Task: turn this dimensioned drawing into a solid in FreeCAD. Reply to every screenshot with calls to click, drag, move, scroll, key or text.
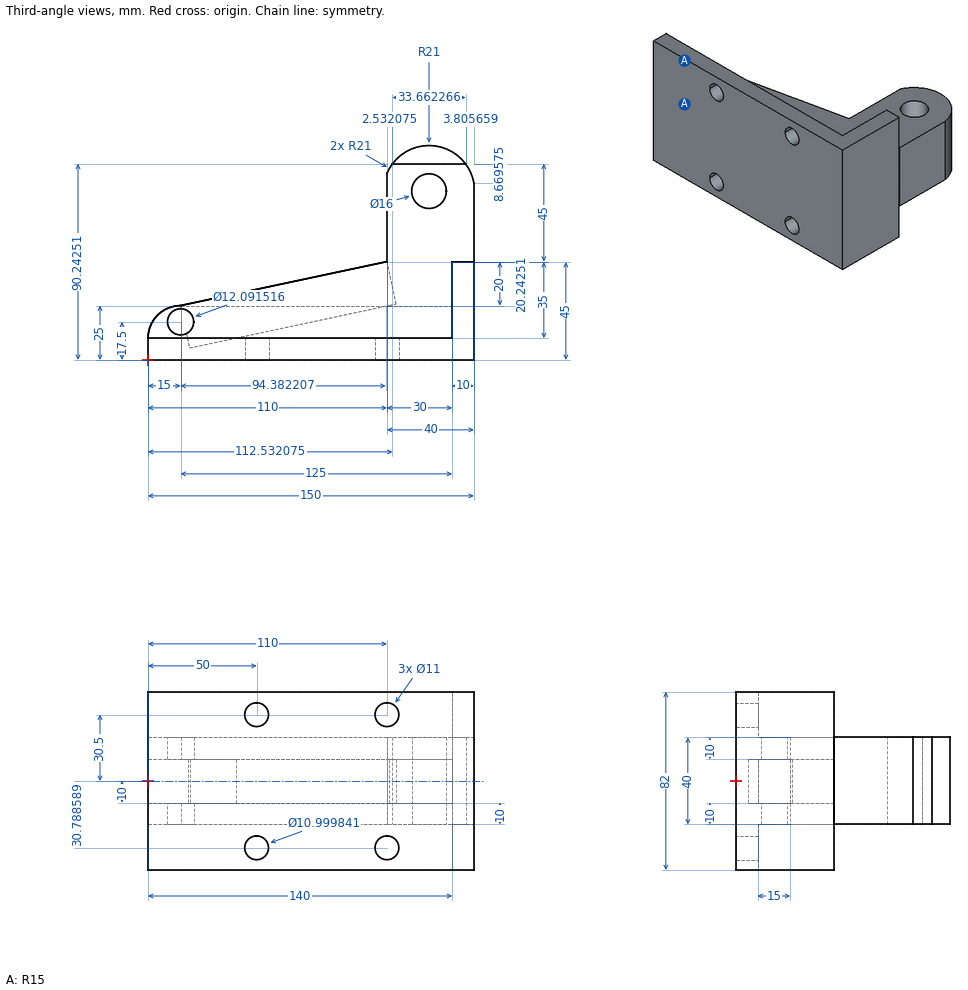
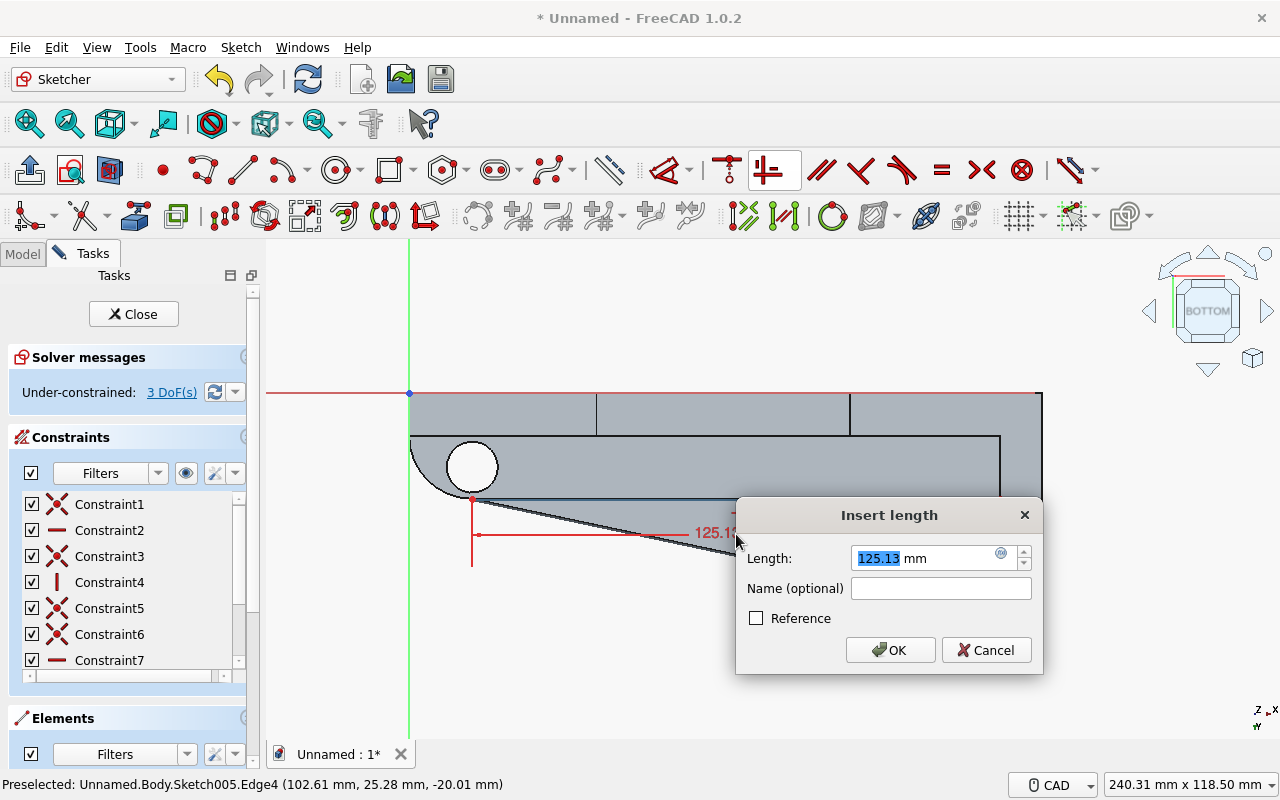
text(125)
key(Return)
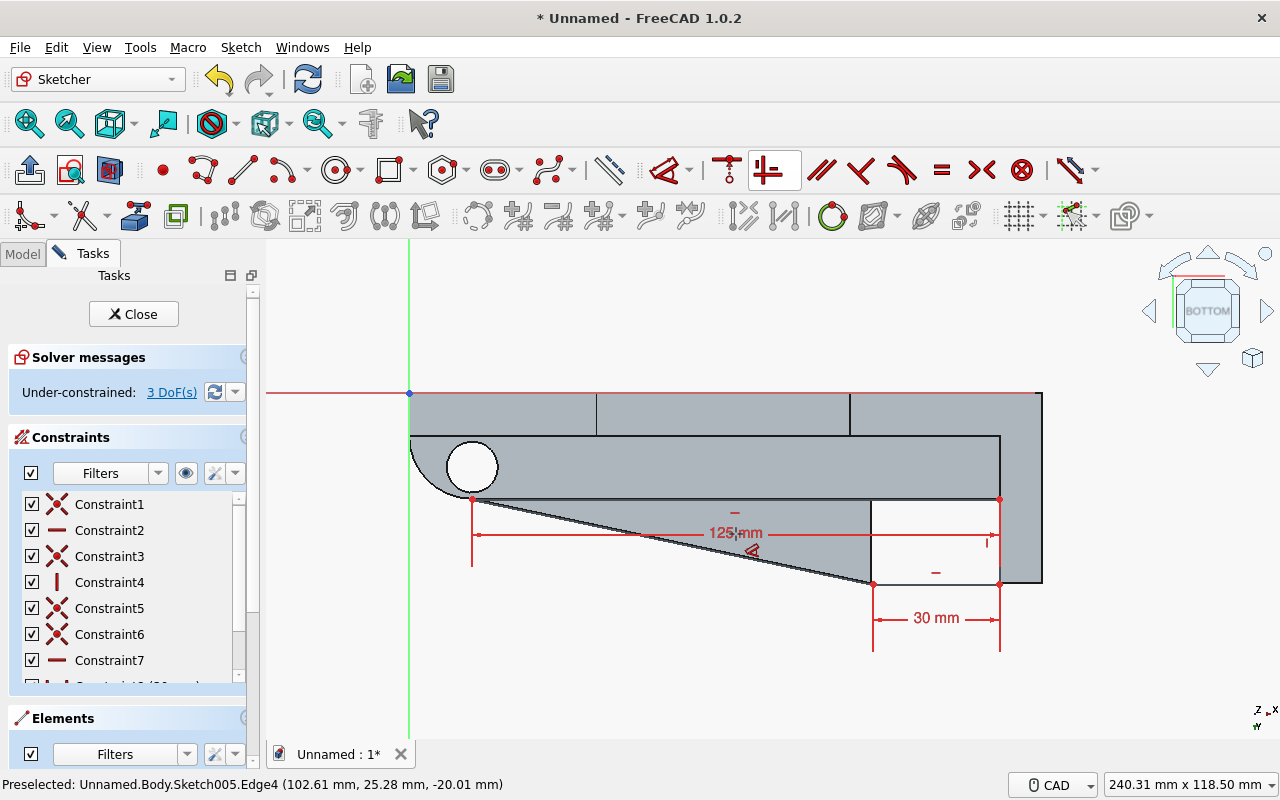
click(472, 500)
click(441, 359)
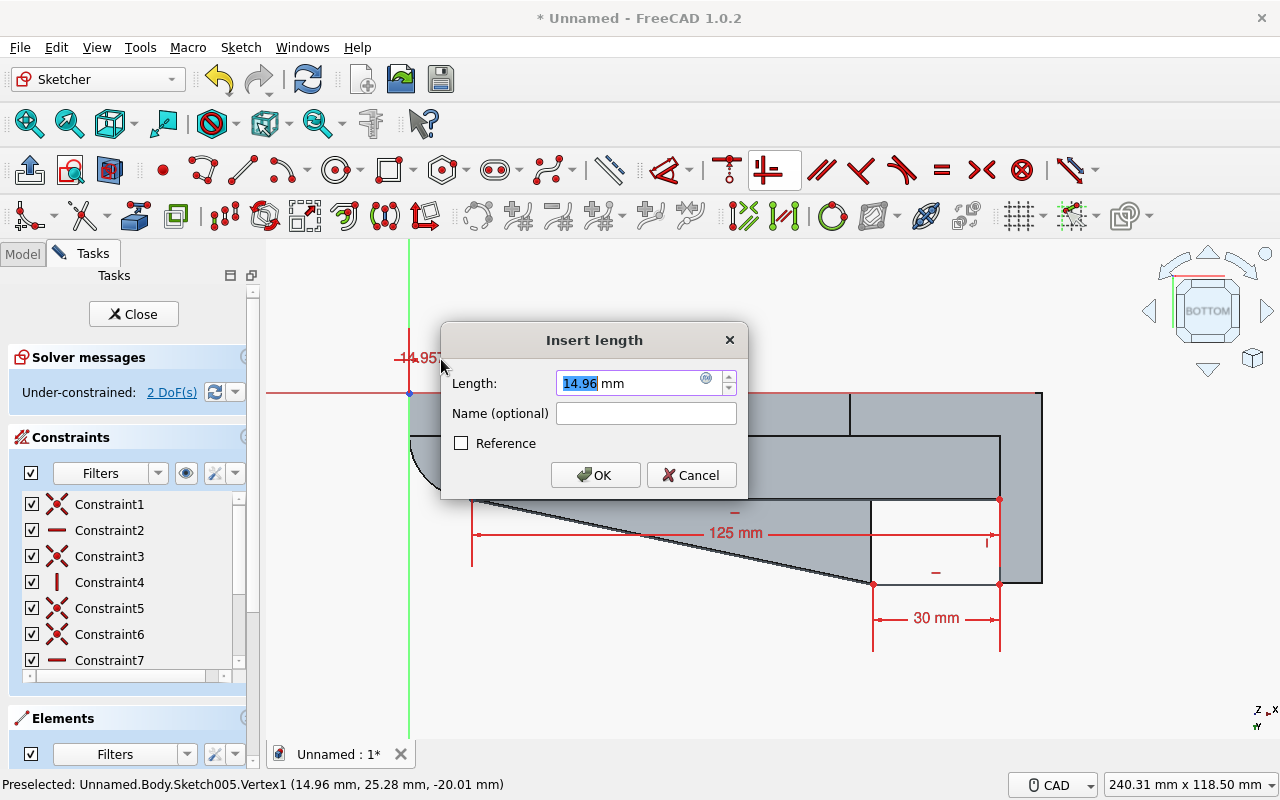
text(15)
key(Return)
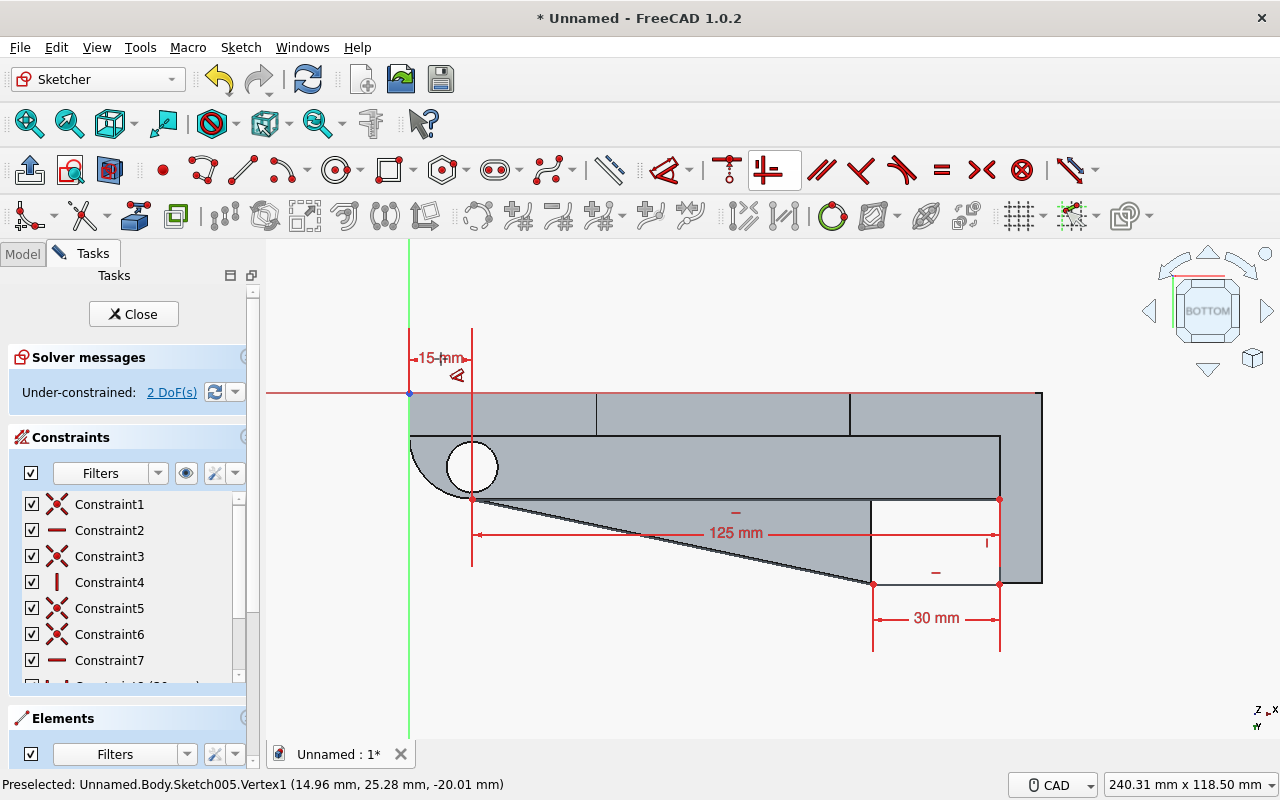
click(472, 500)
click(375, 447)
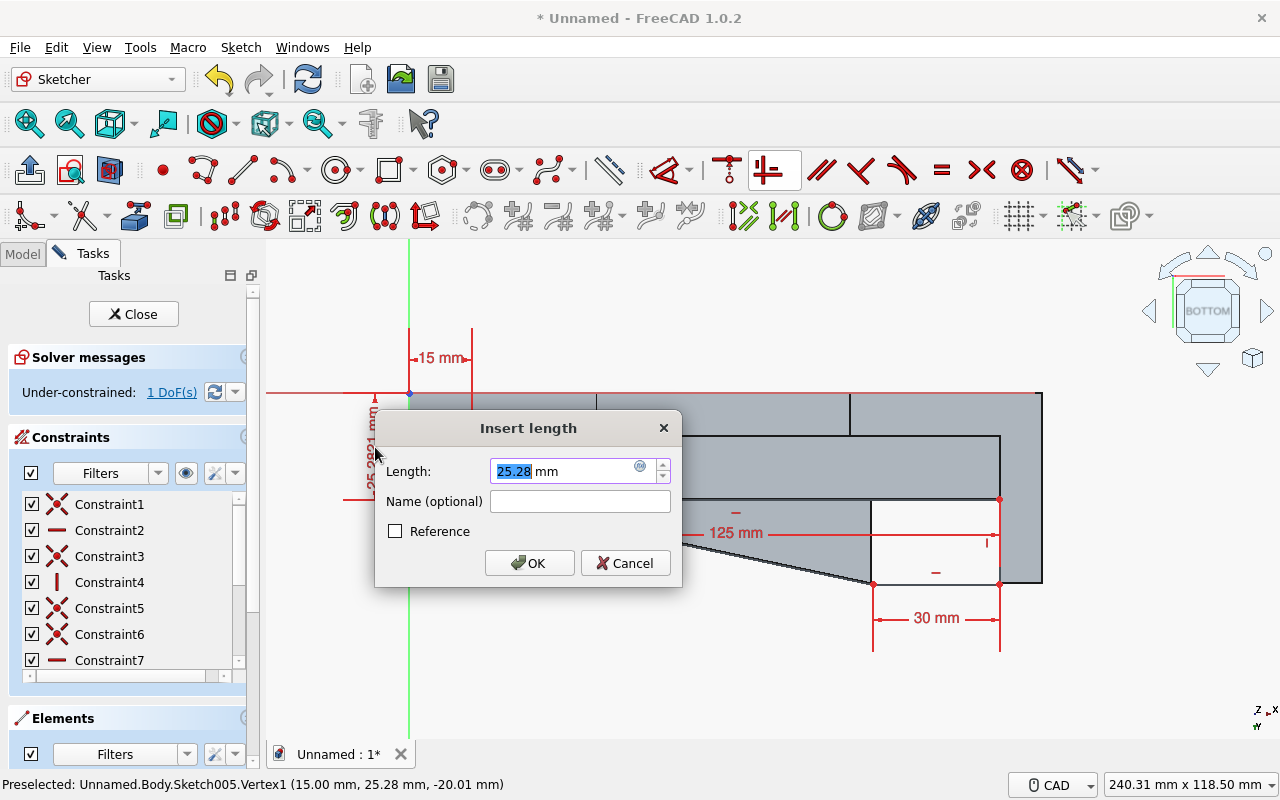
text(25)
key(Return)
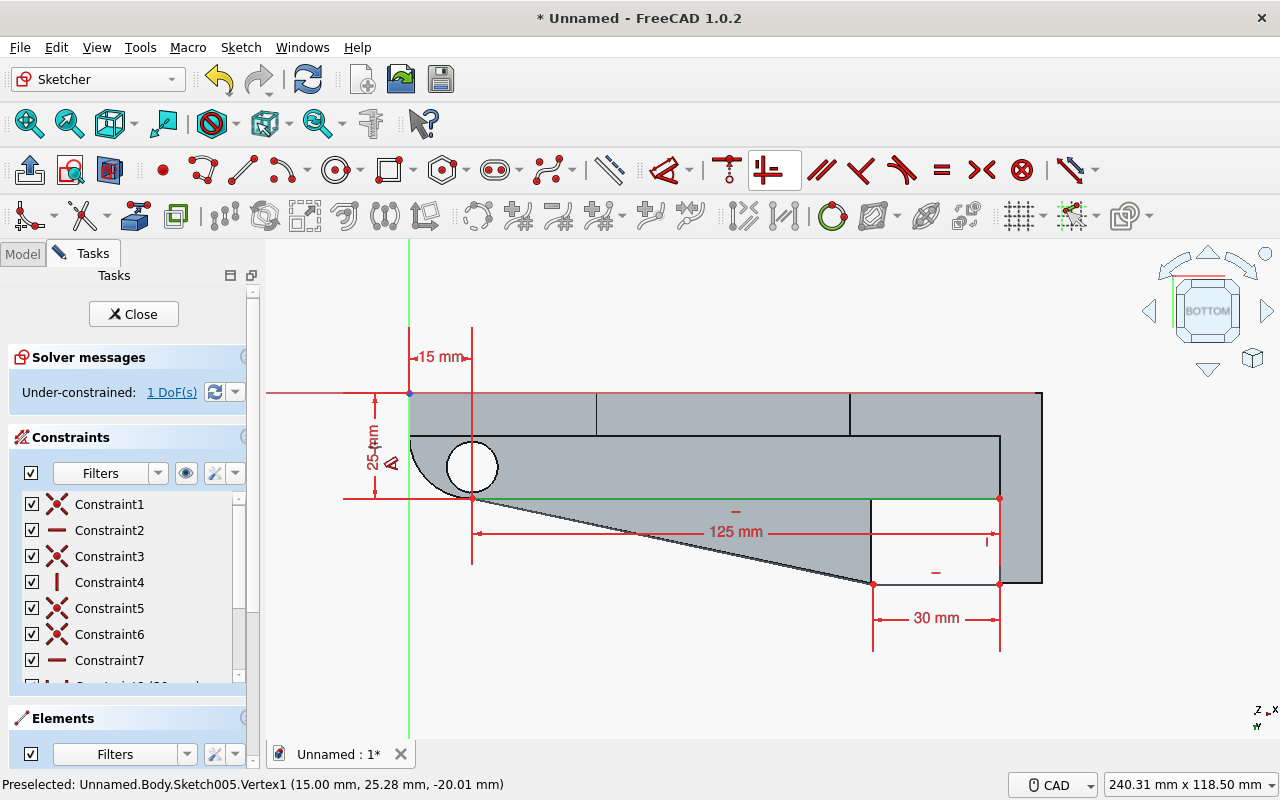
click(1000, 559)
click(1034, 542)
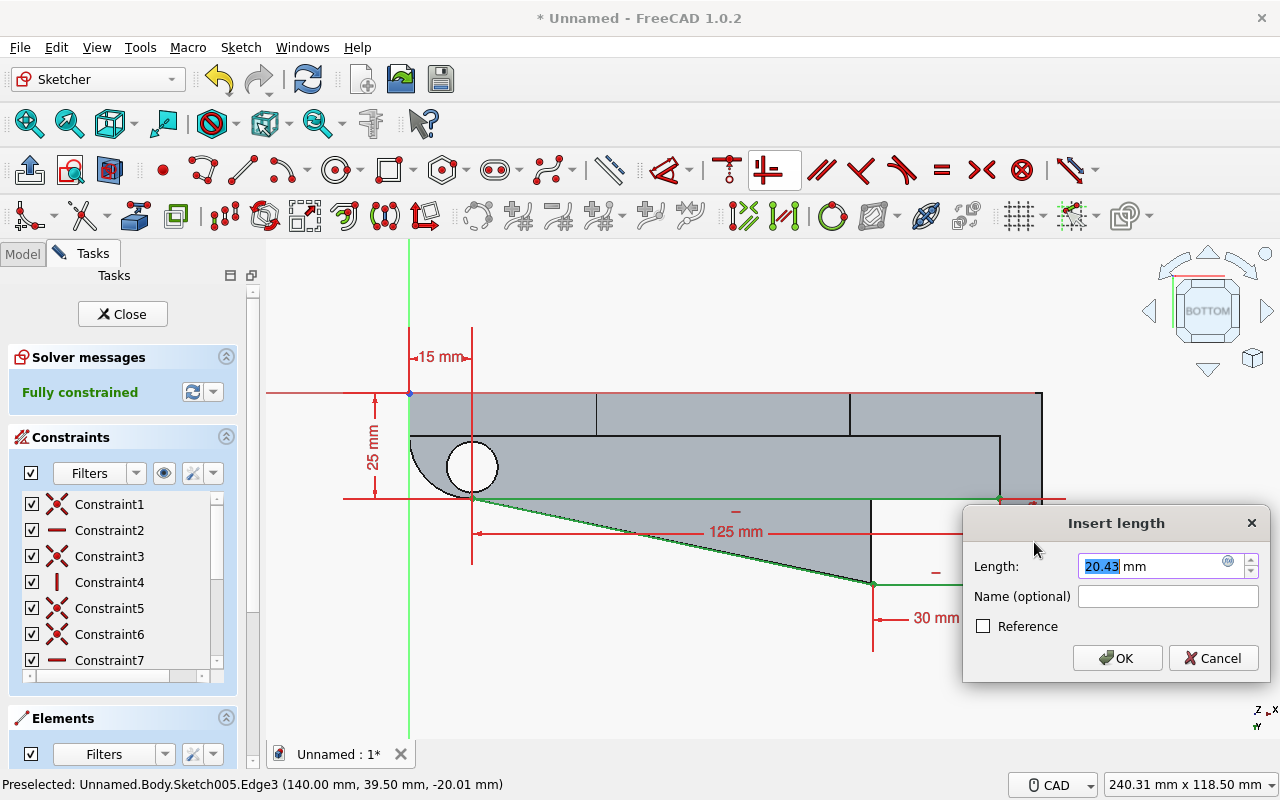
text(20.24251)
key(Return)
key(Escape)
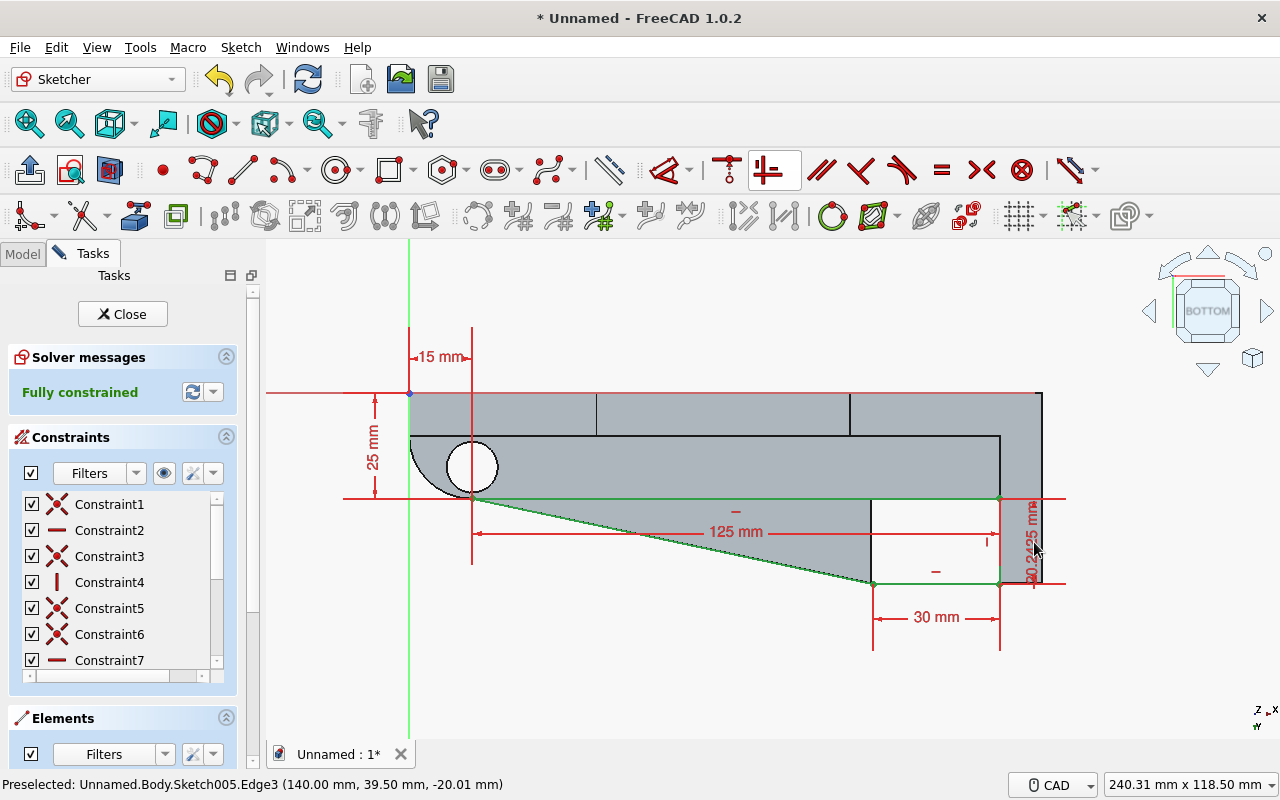
click(123, 314)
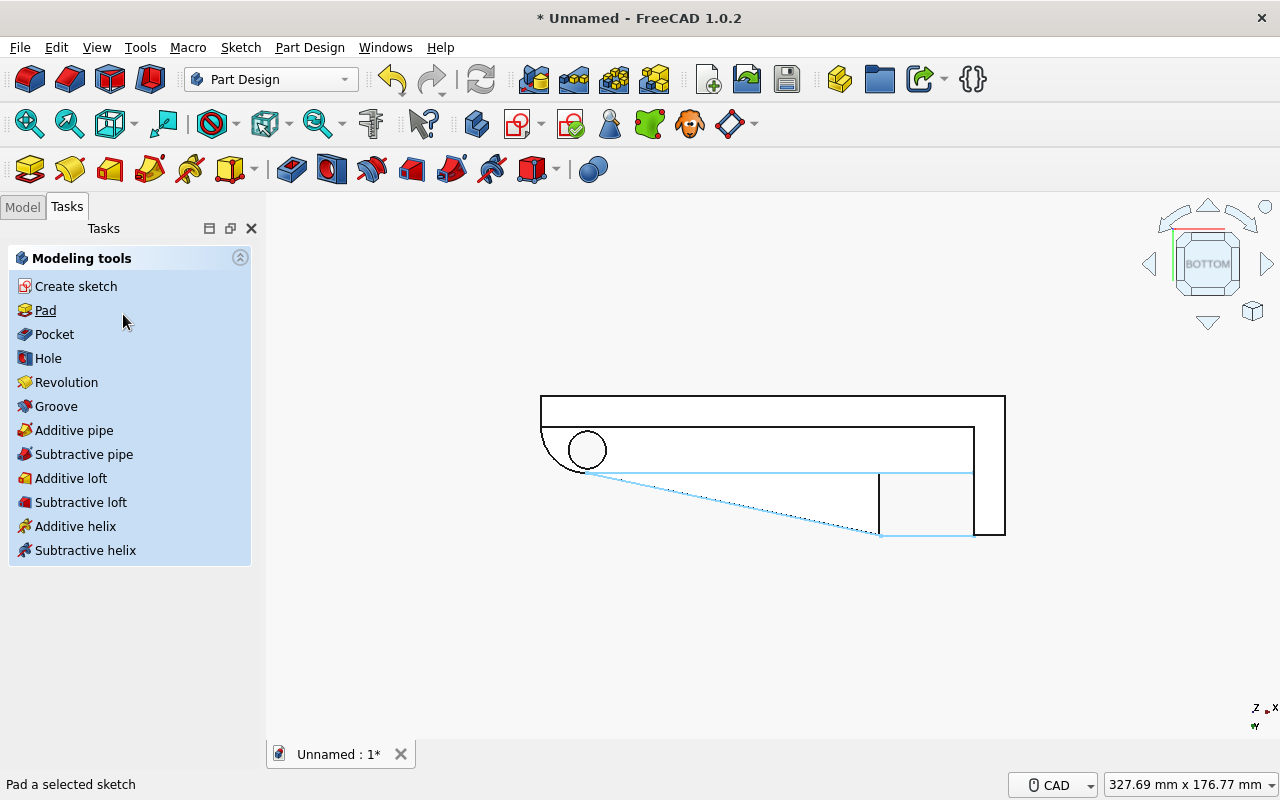
click(30, 170)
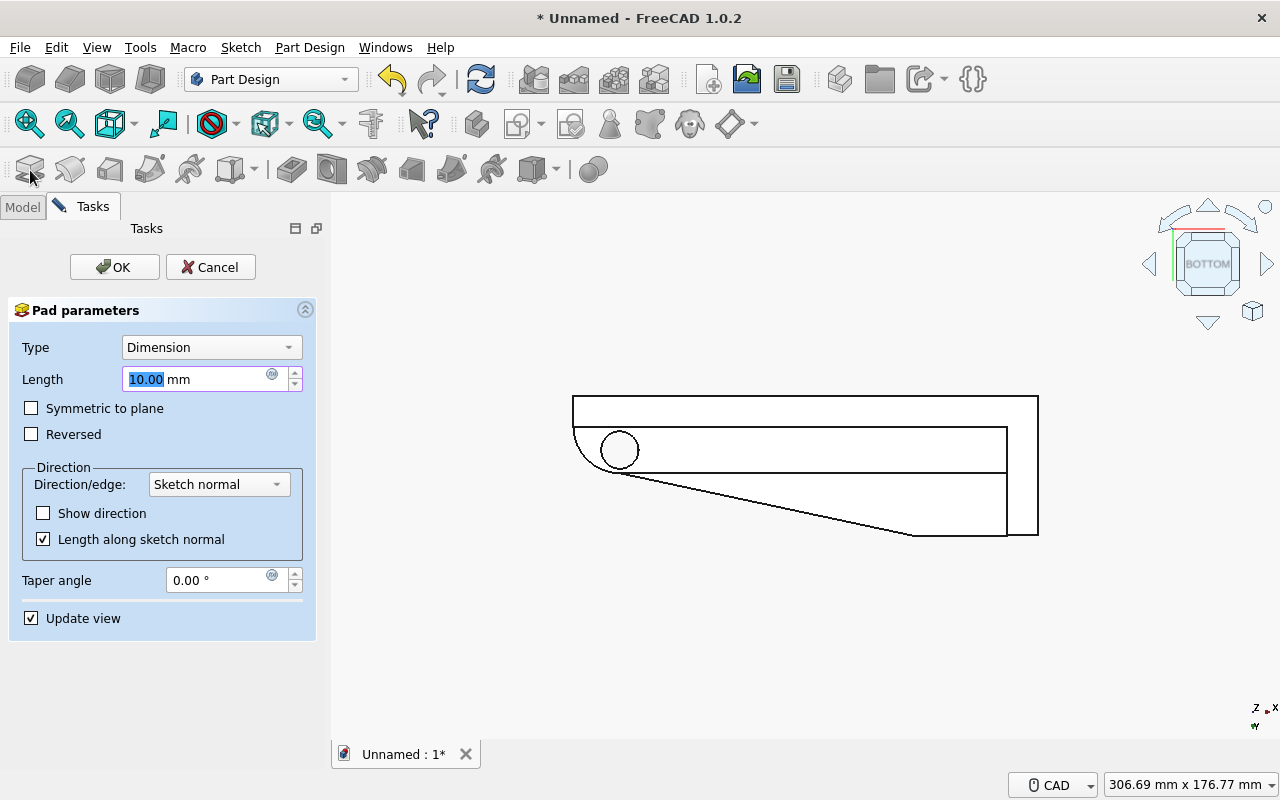
text(10)
key(Tab)